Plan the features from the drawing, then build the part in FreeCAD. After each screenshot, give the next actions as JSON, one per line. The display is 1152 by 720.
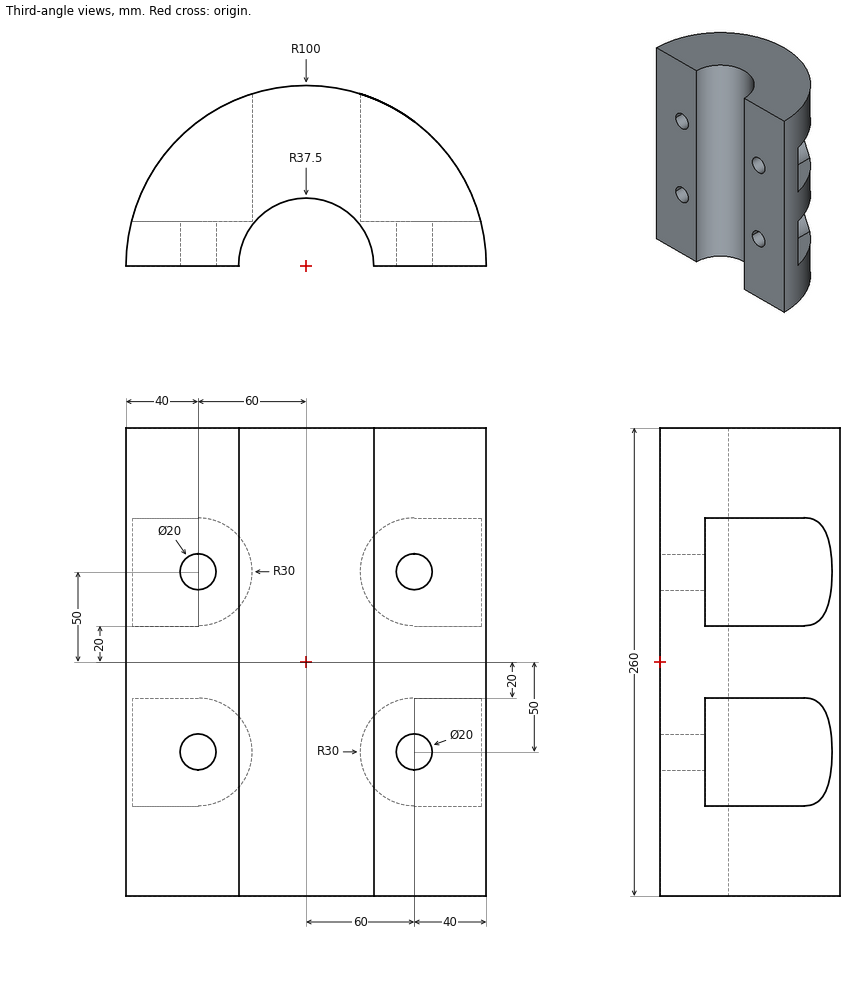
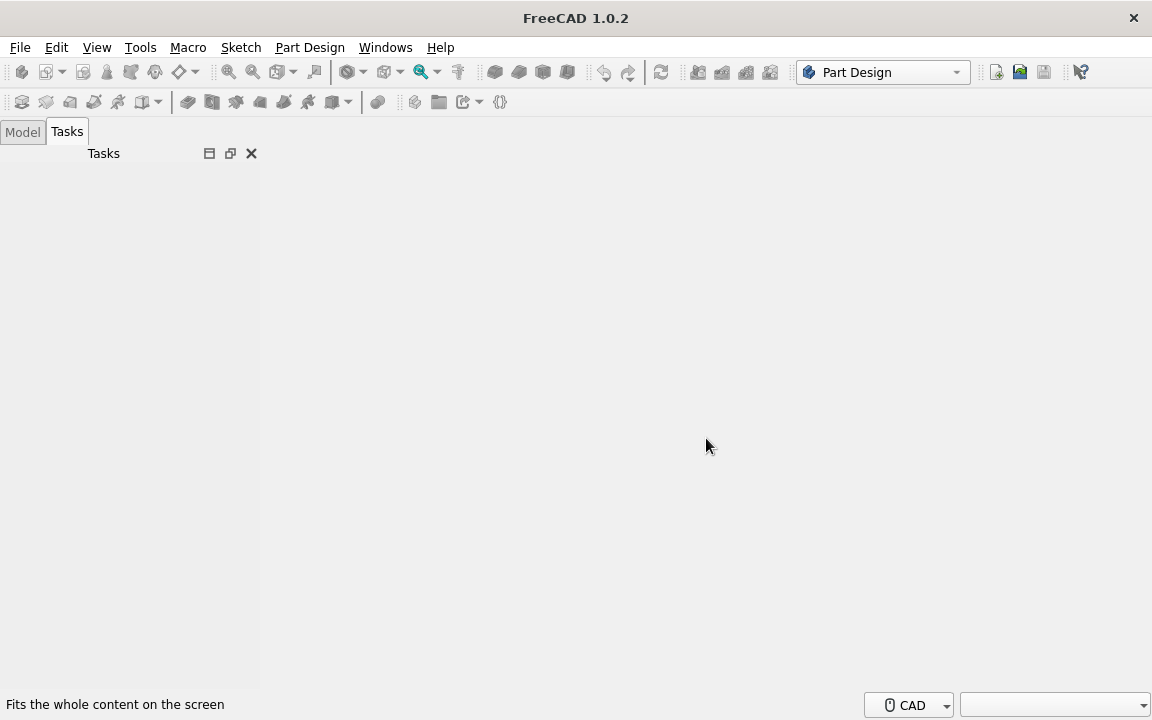
{"action": "key", "text": "ctrl+n"}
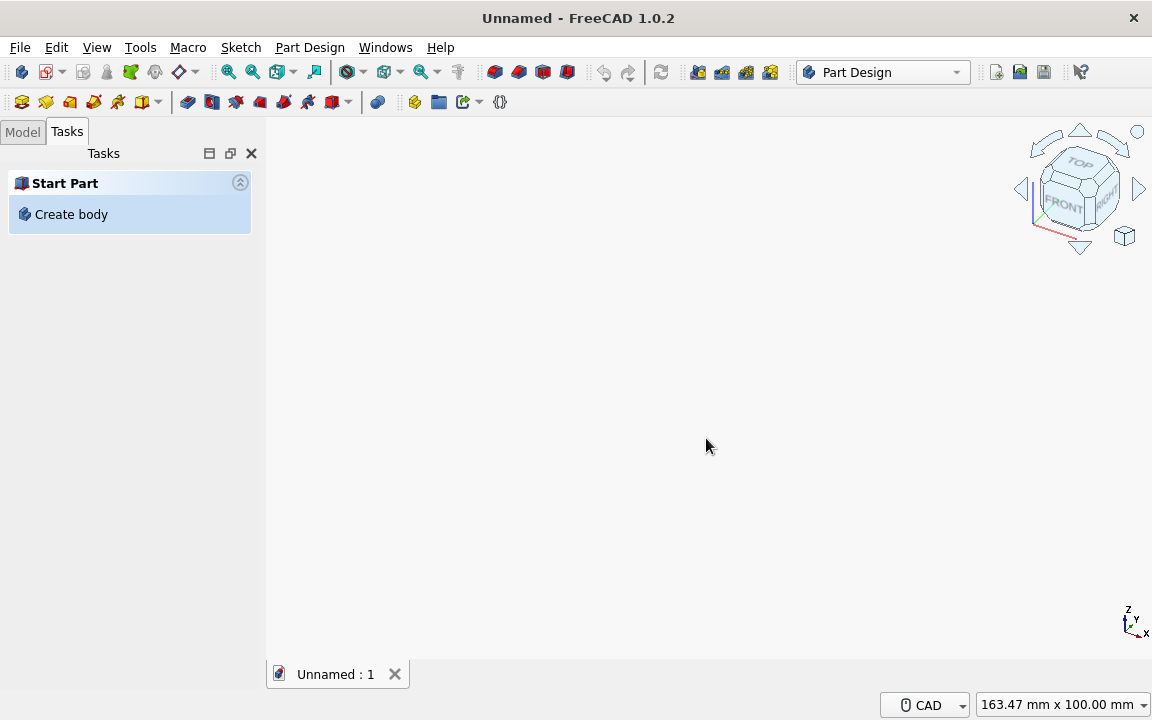
{"action": "left_click", "coordinate": [46, 72]}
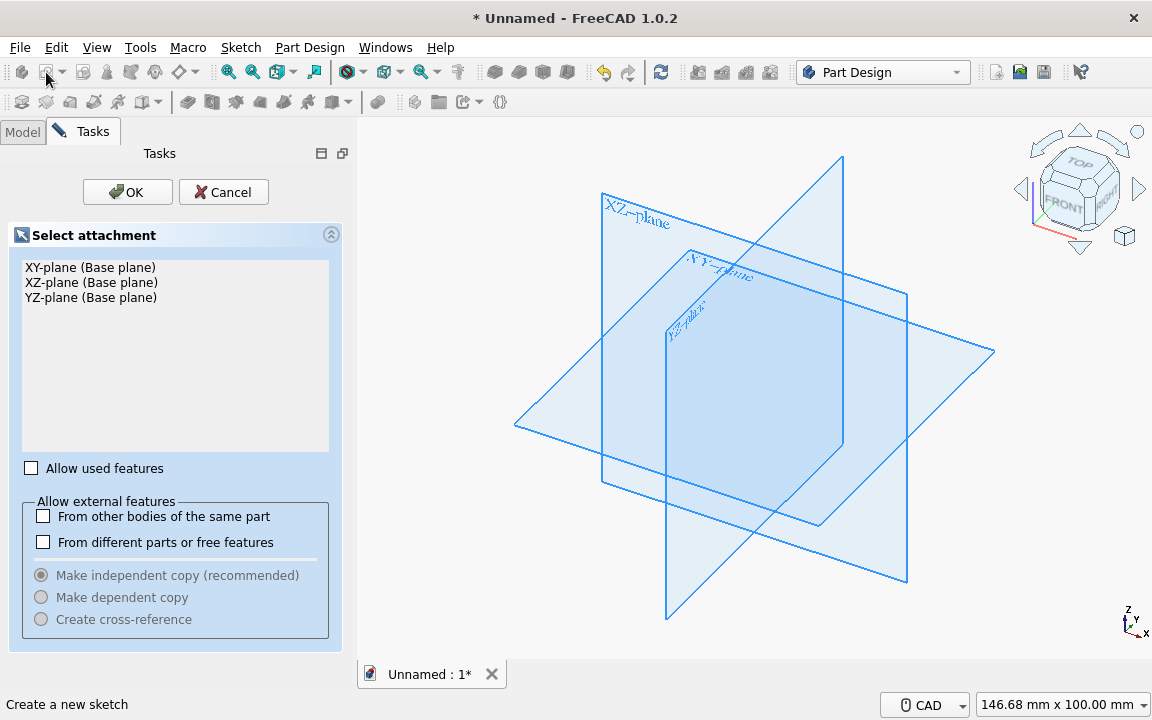
{"action": "left_click", "coordinate": [82, 268]}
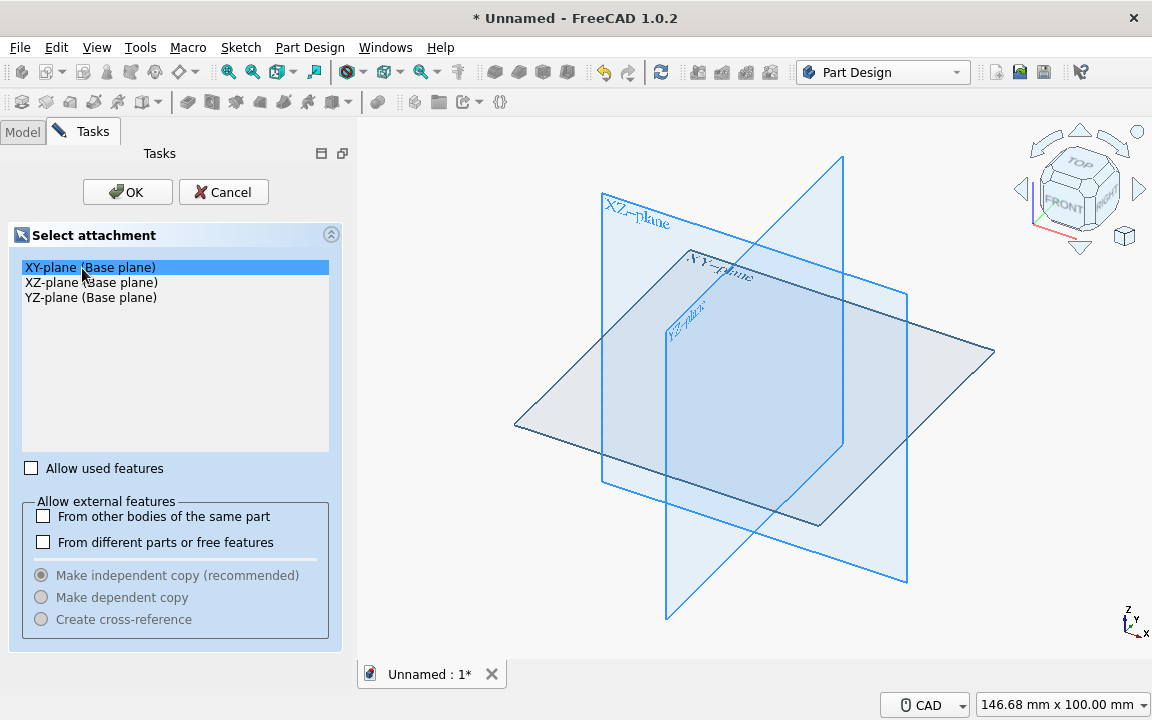
{"action": "left_click", "coordinate": [128, 192]}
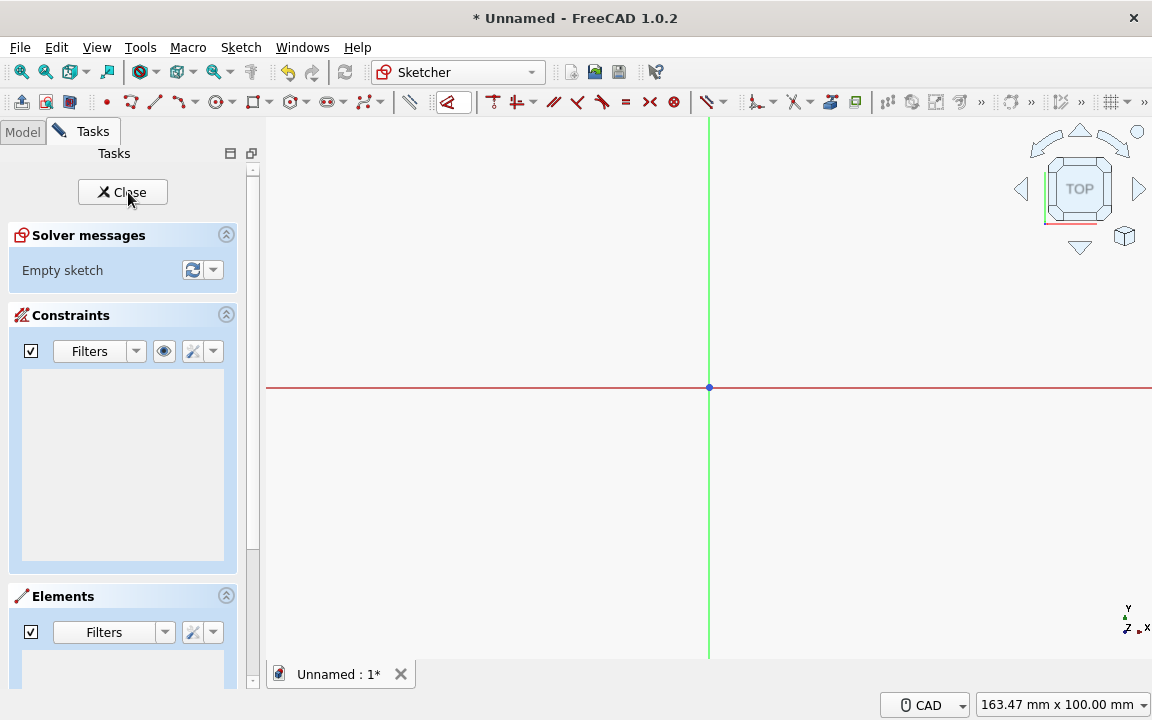
{"action": "scroll", "coordinate": [585, 609], "scroll_direction": "down", "scroll_amount": 4}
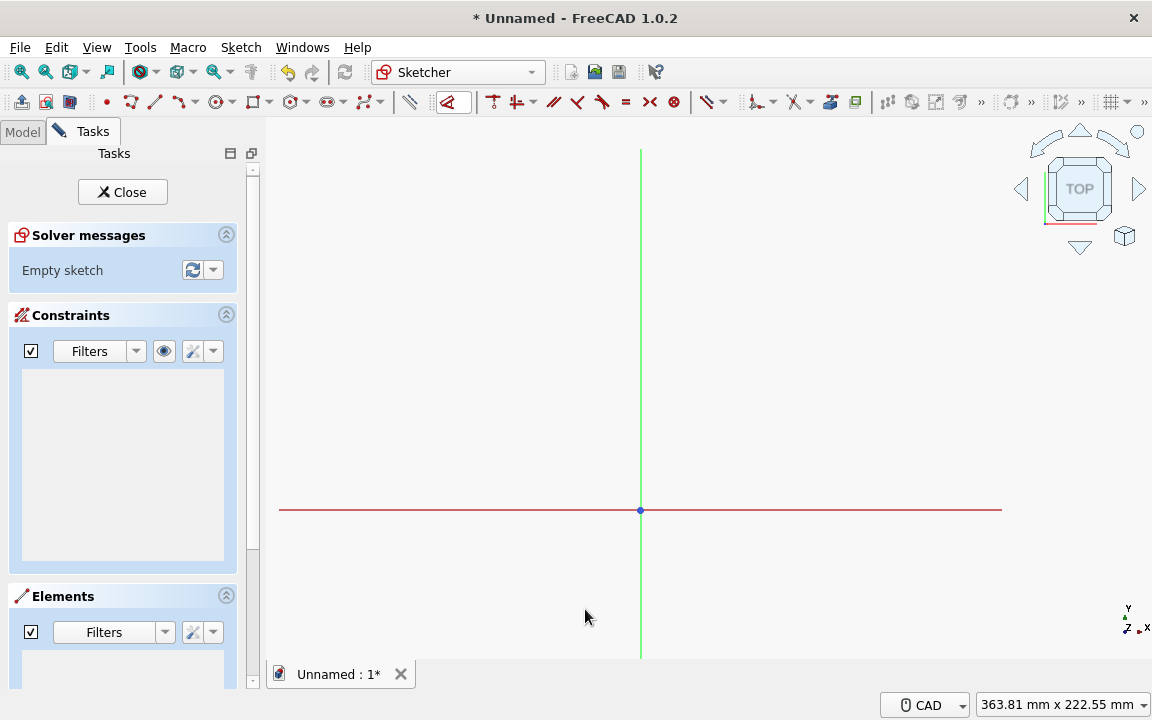
{"action": "left_click", "coordinate": [156, 102]}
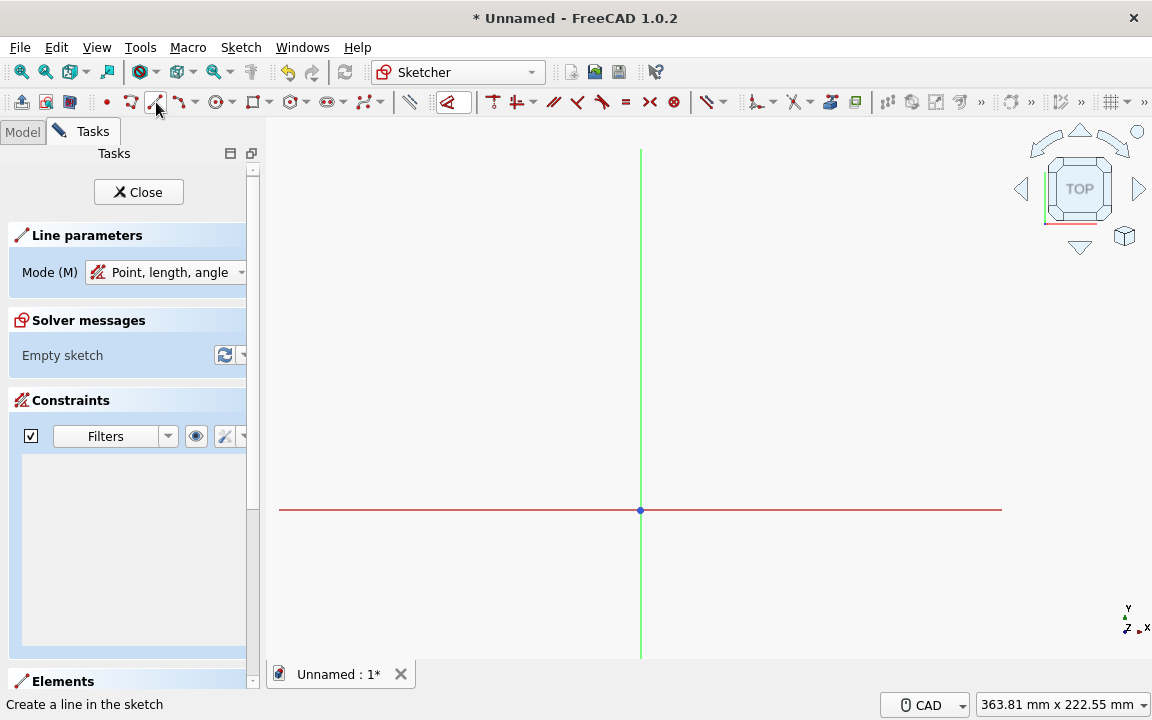
{"action": "left_click", "coordinate": [397, 510]}
{"action": "left_click", "coordinate": [550, 501]}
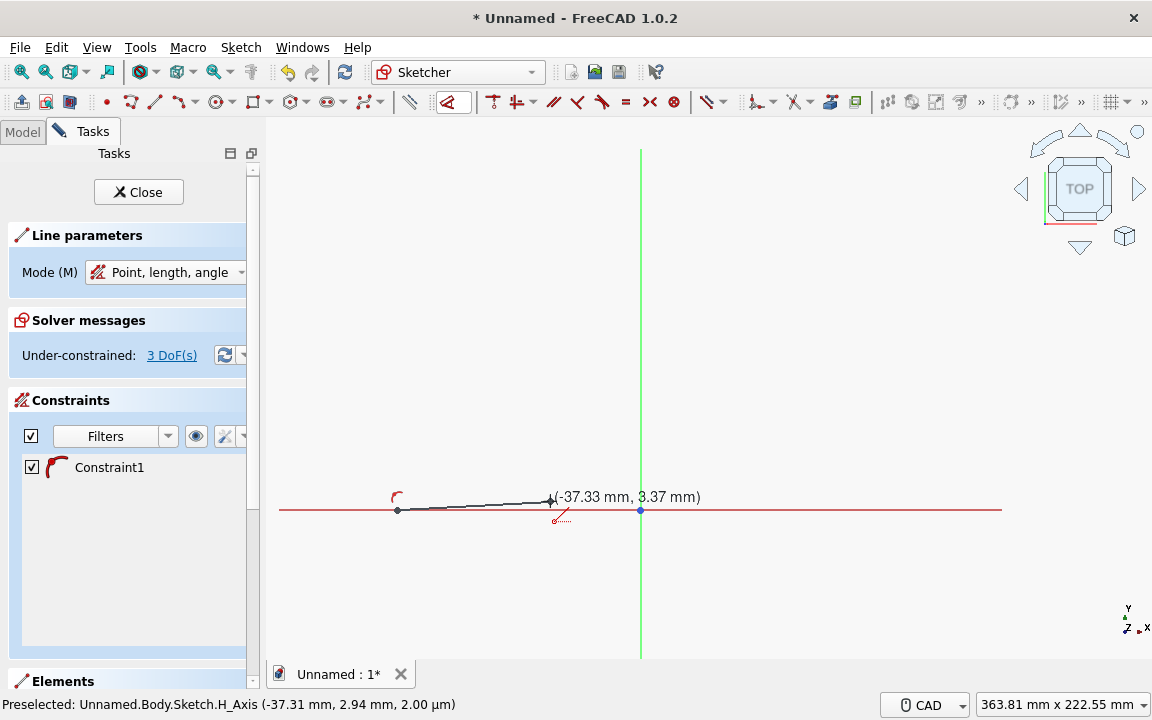
{"action": "left_click", "coordinate": [732, 510]}
{"action": "left_click", "coordinate": [884, 501]}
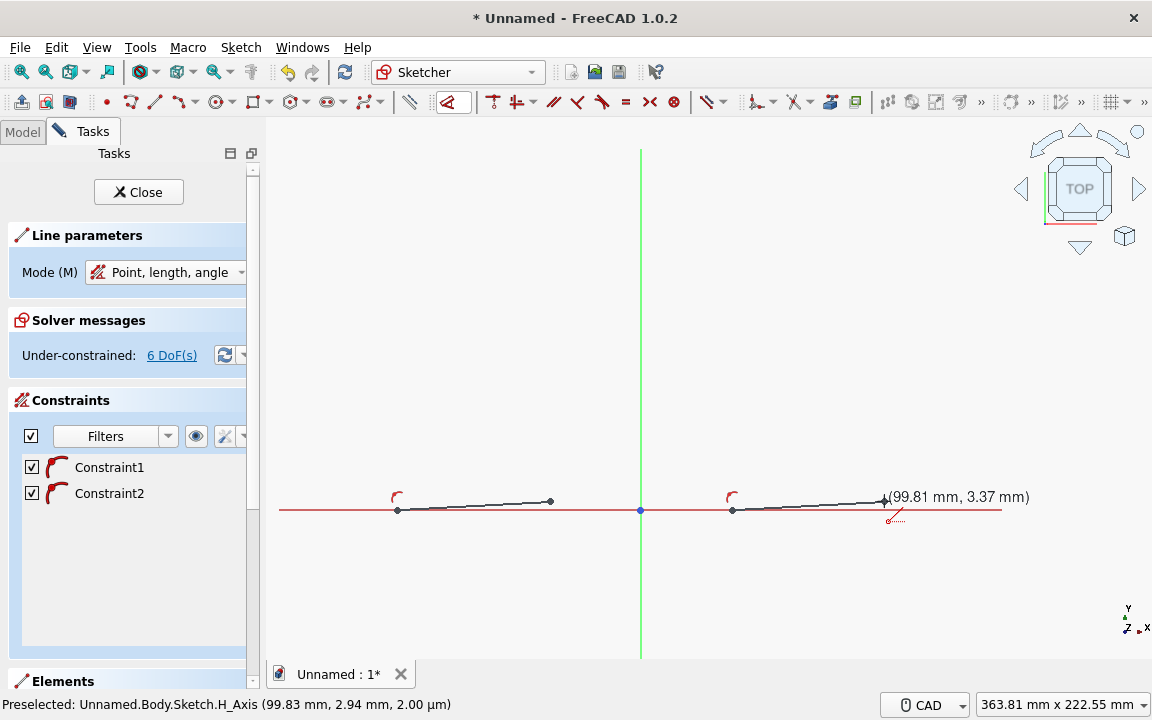
{"action": "key", "text": "g 3 a"}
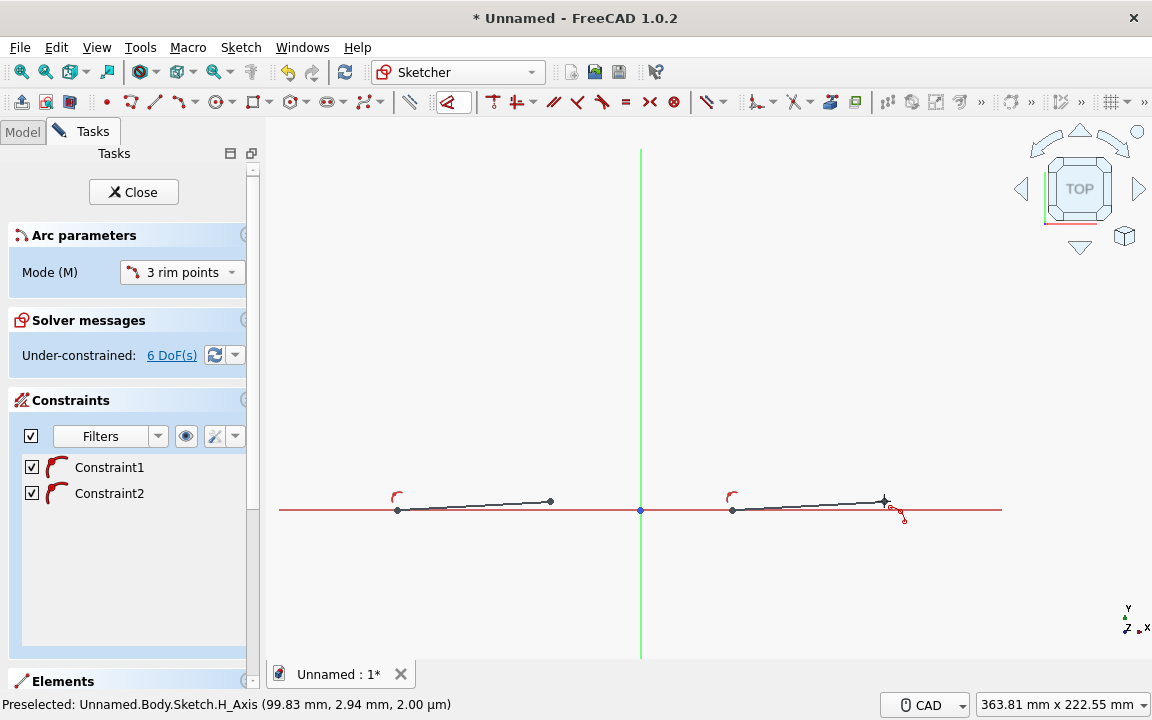
{"action": "left_click", "coordinate": [550, 502]}
{"action": "left_click", "coordinate": [732, 510]}
{"action": "left_click", "coordinate": [669, 423]}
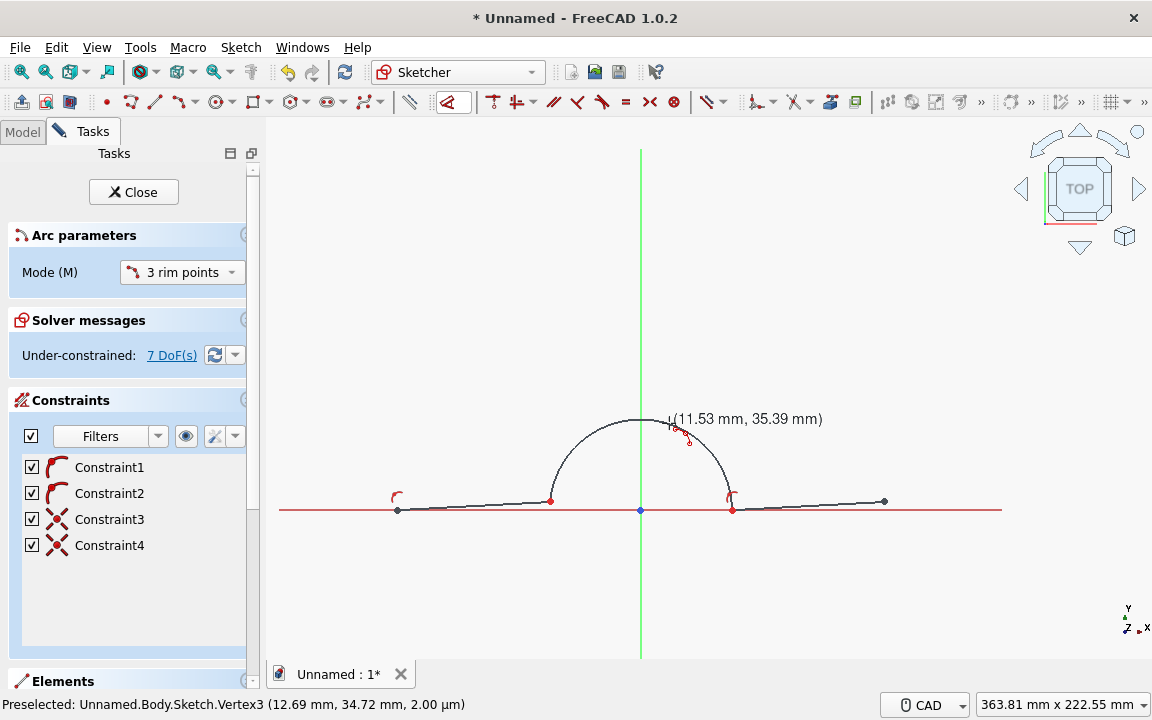
{"action": "left_click", "coordinate": [884, 502]}
{"action": "left_click", "coordinate": [397, 510]}
{"action": "left_click", "coordinate": [716, 279]}
{"action": "key", "text": "Escape"}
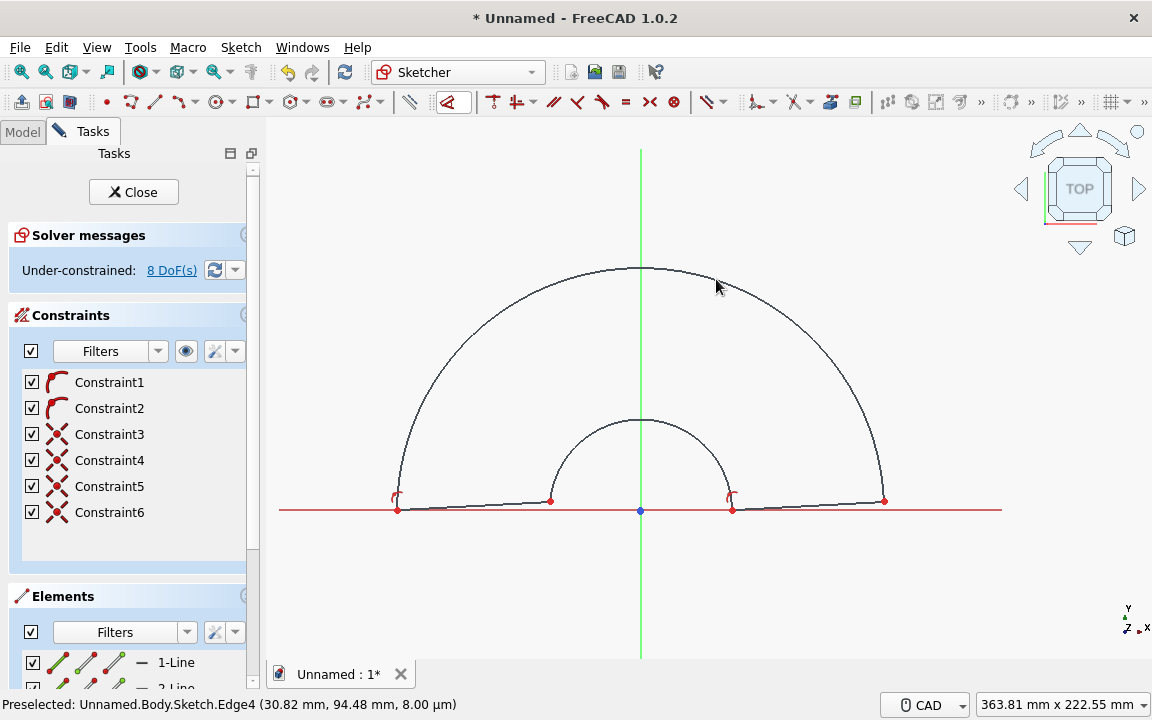
{"action": "left_click", "coordinate": [443, 508]}